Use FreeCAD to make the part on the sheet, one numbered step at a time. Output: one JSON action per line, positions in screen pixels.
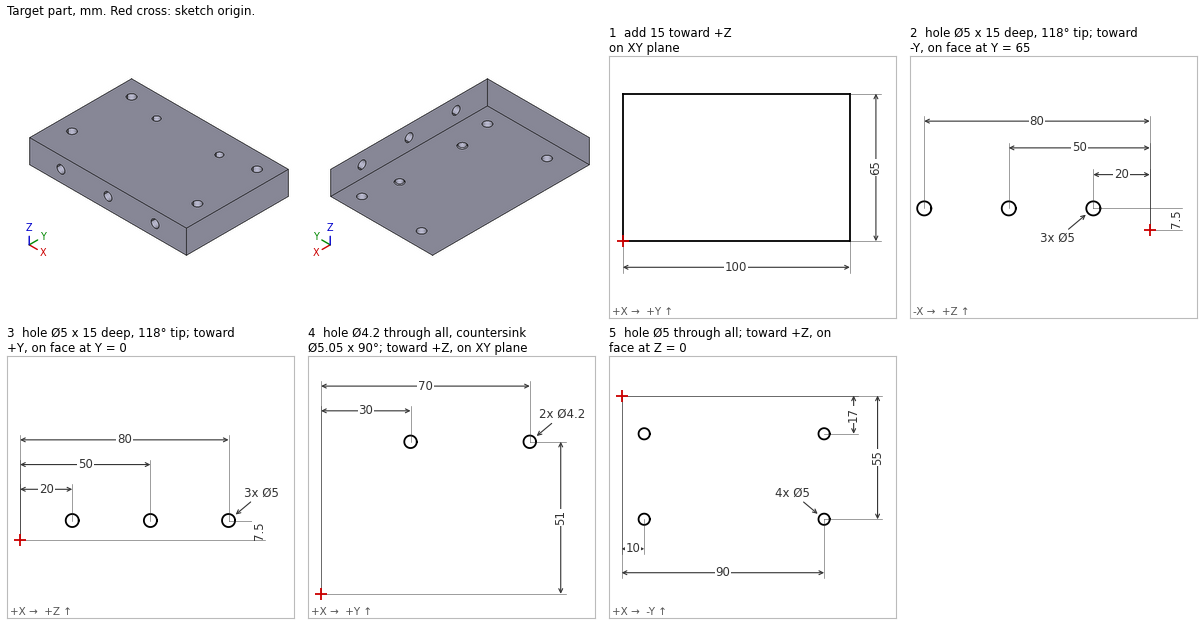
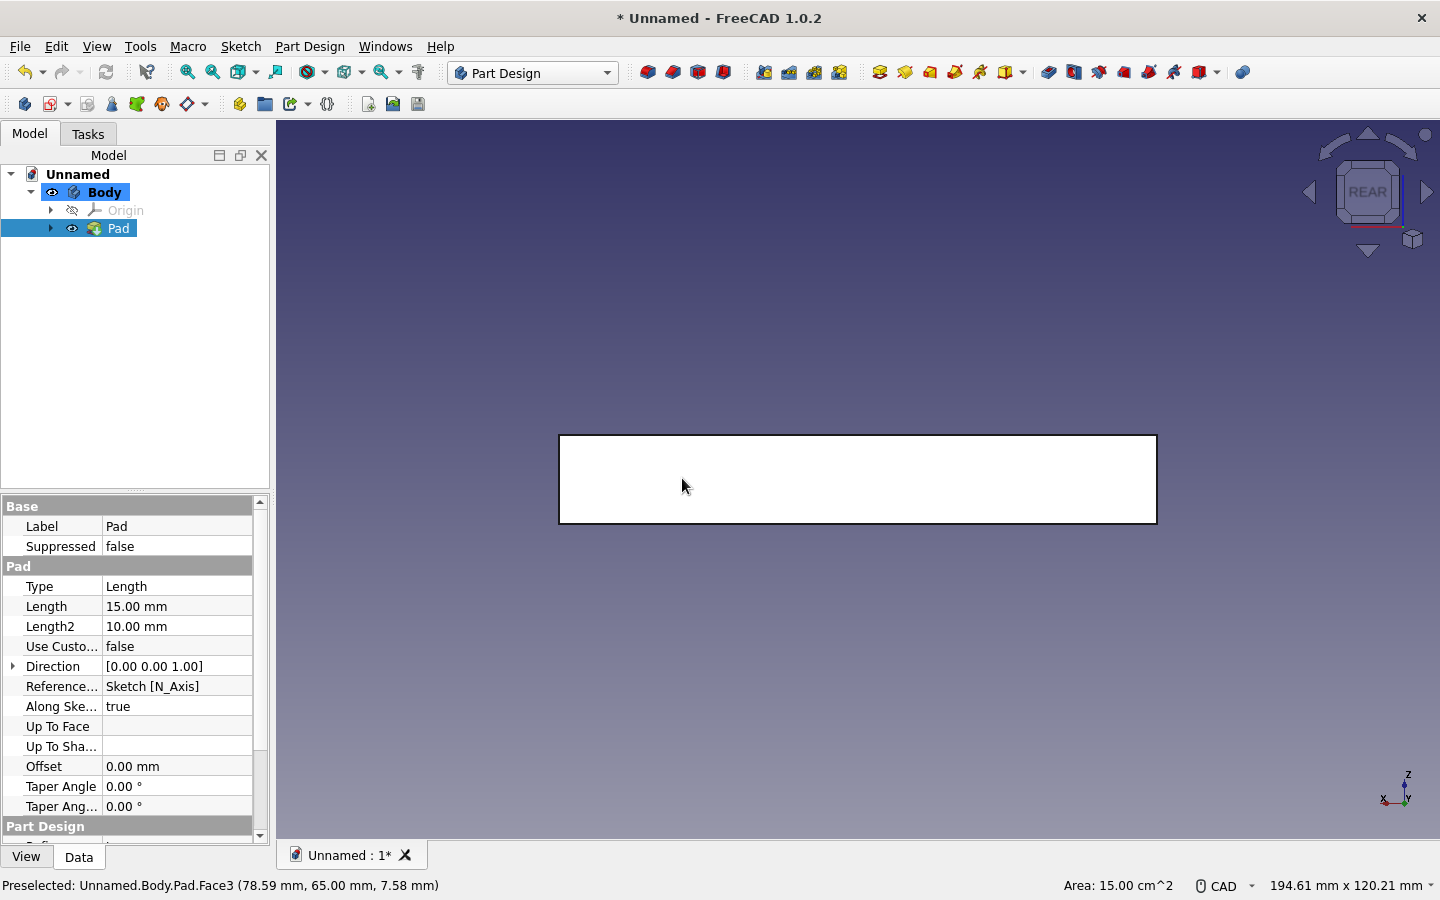
{"action": "left_click", "coordinate": [50, 104]}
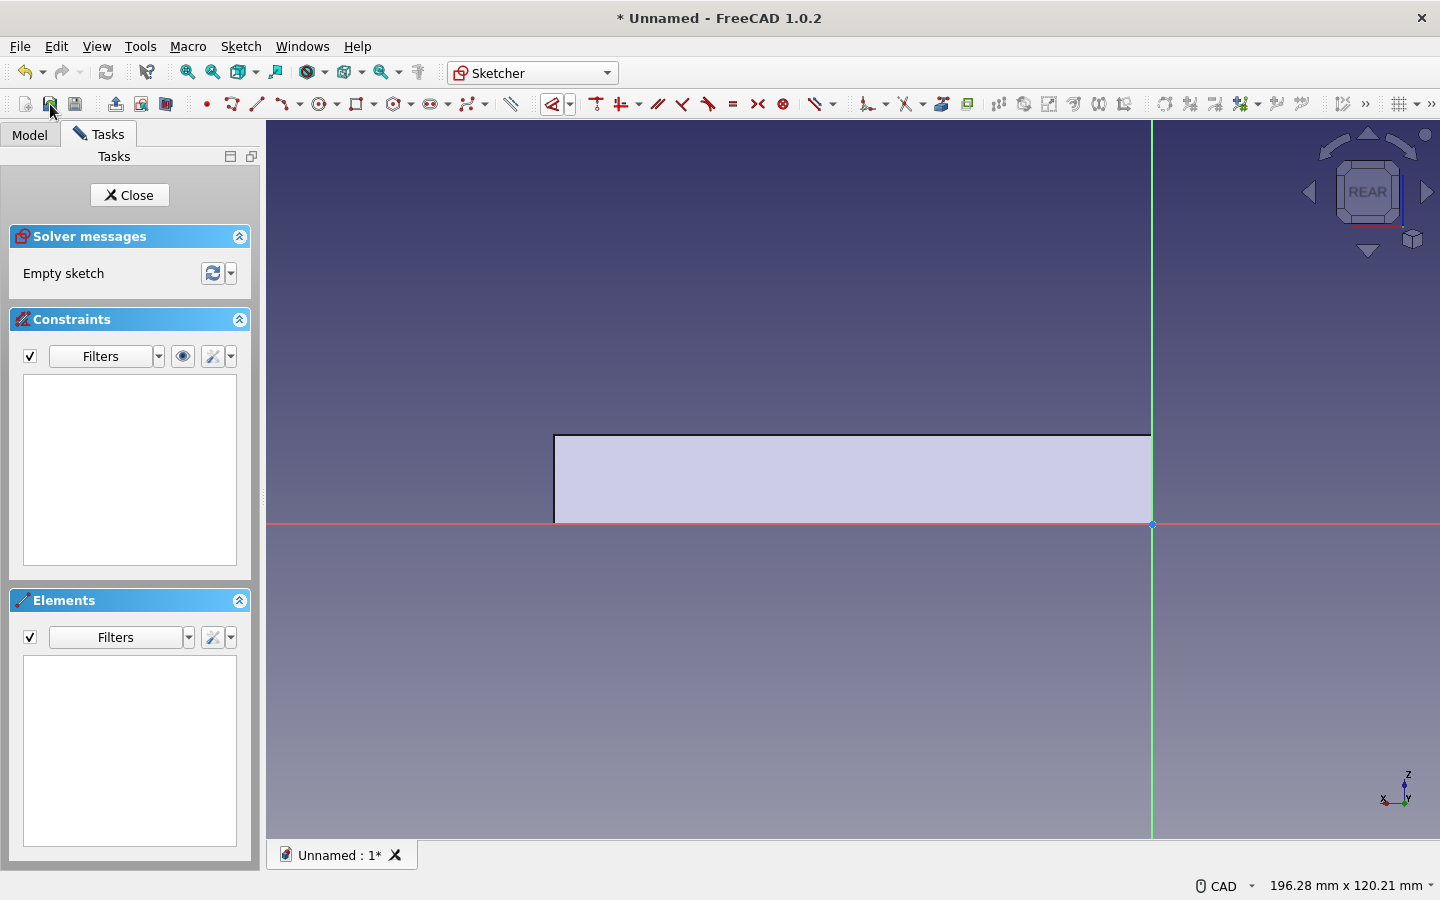
{"action": "scroll", "coordinate": [1151, 525], "scroll_direction": "up", "scroll_amount": 2}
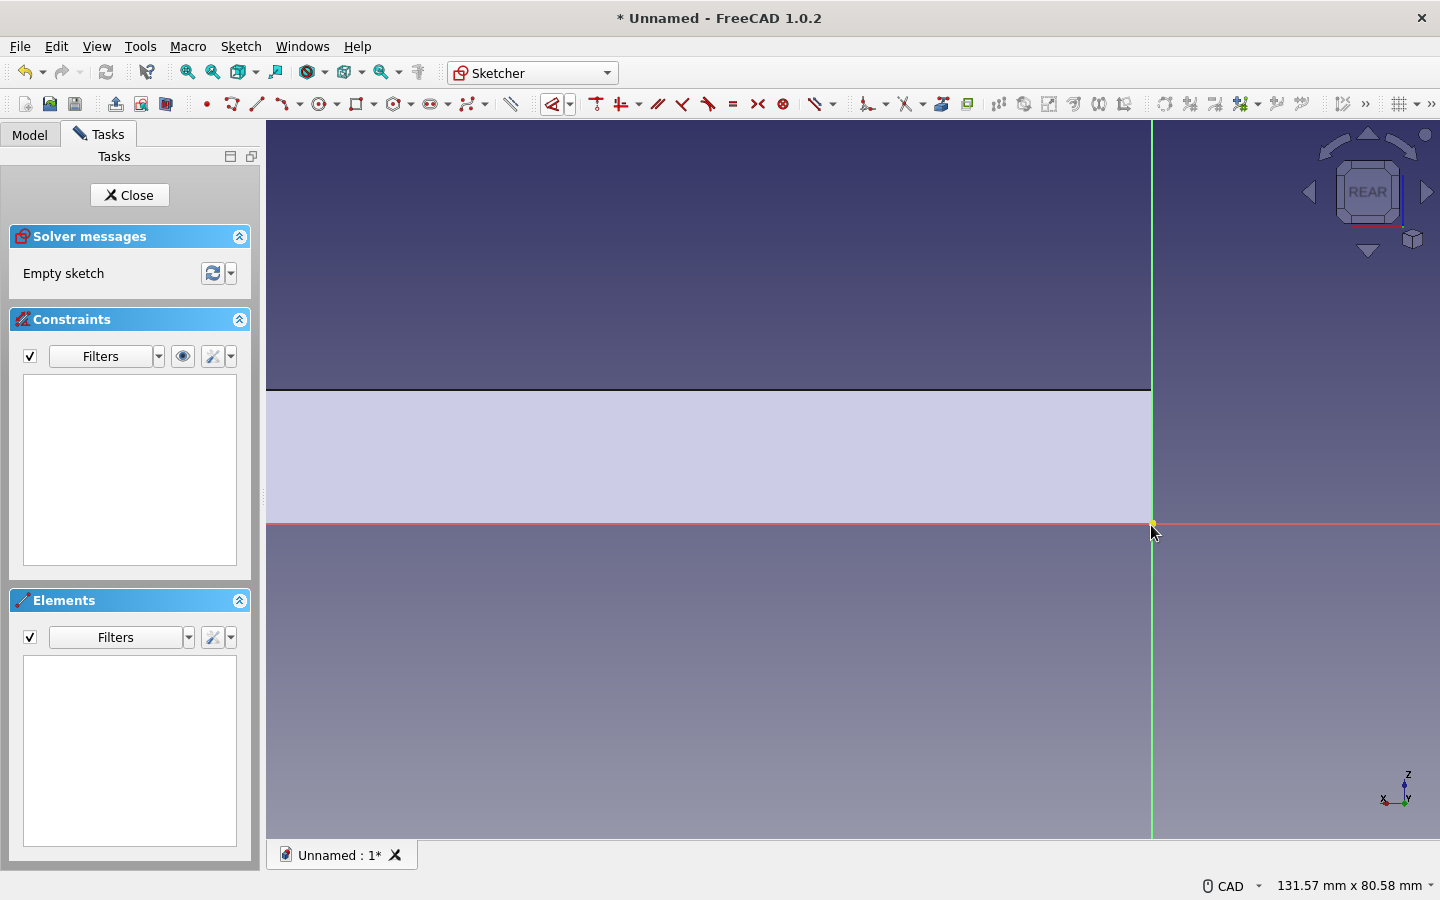
{"action": "left_click", "coordinate": [318, 104]}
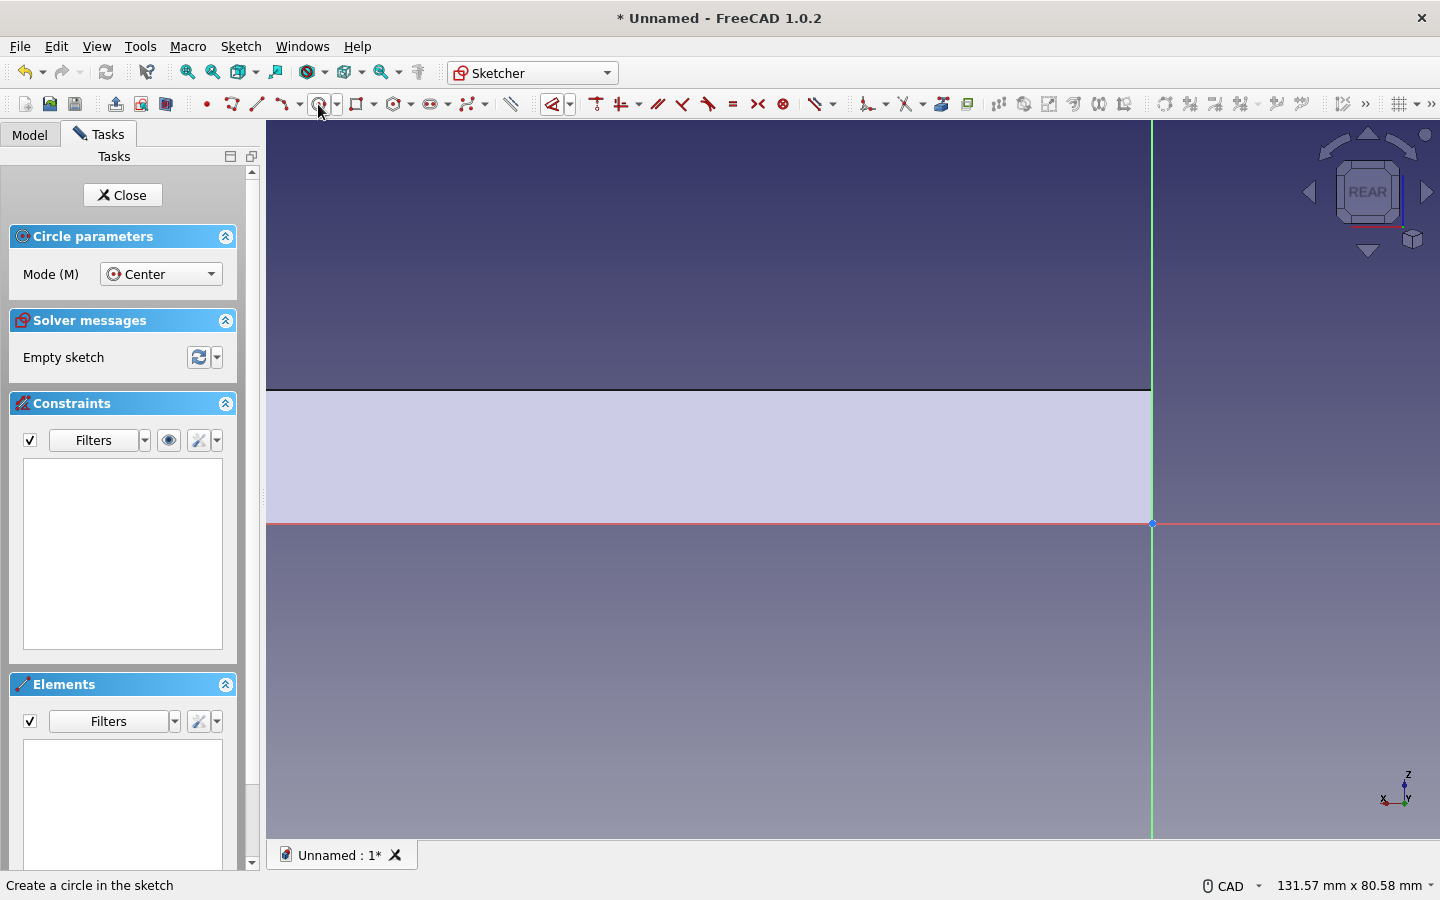
{"action": "left_click", "coordinate": [974, 457]}
{"action": "mouse_move", "coordinate": [990, 441]}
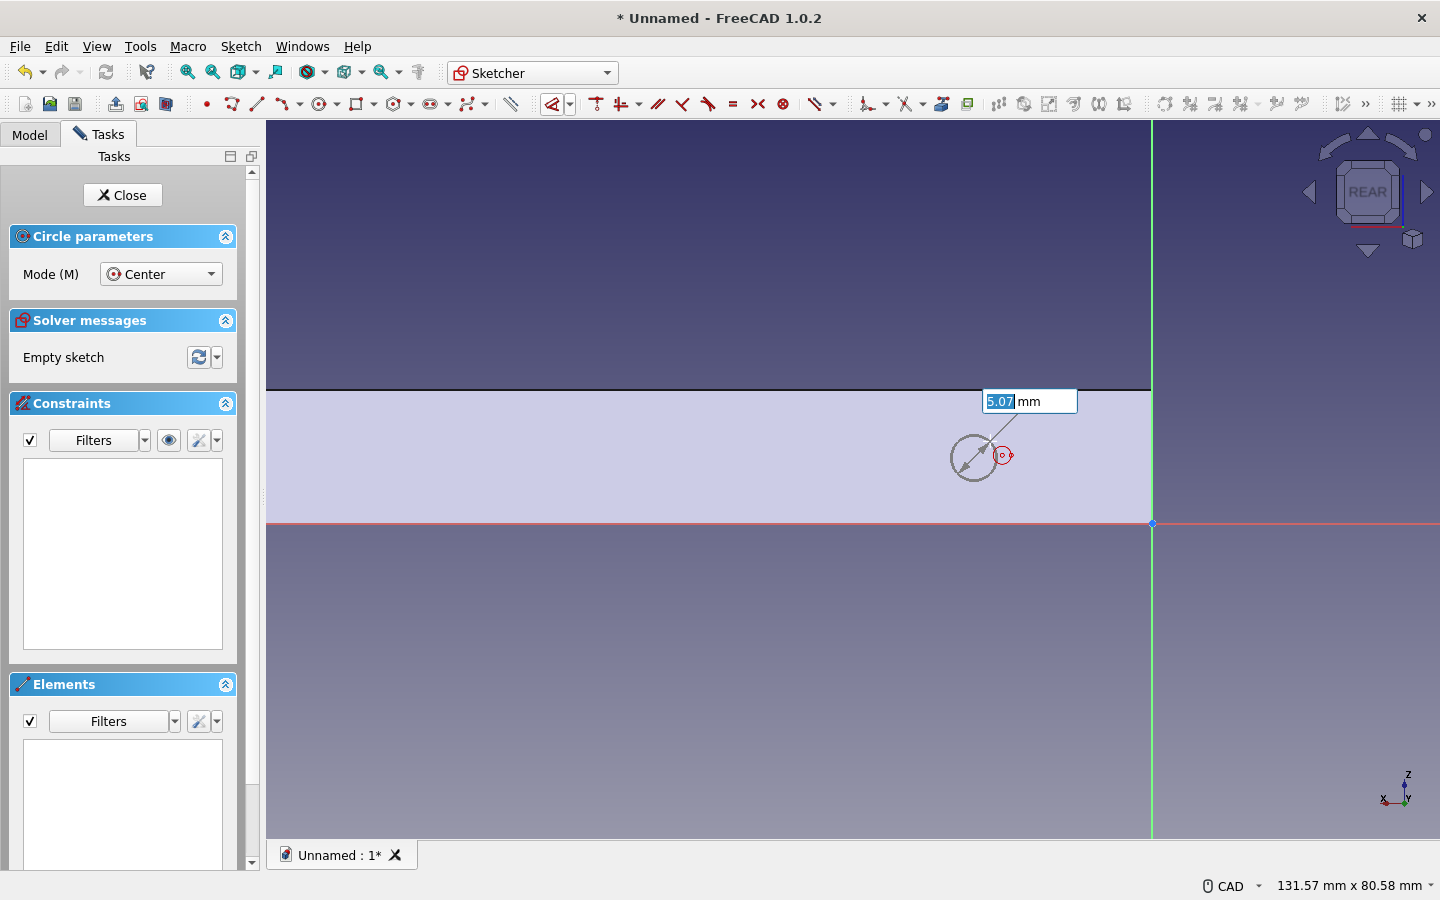
{"action": "type", "text": "5"}
{"action": "key", "text": "Return"}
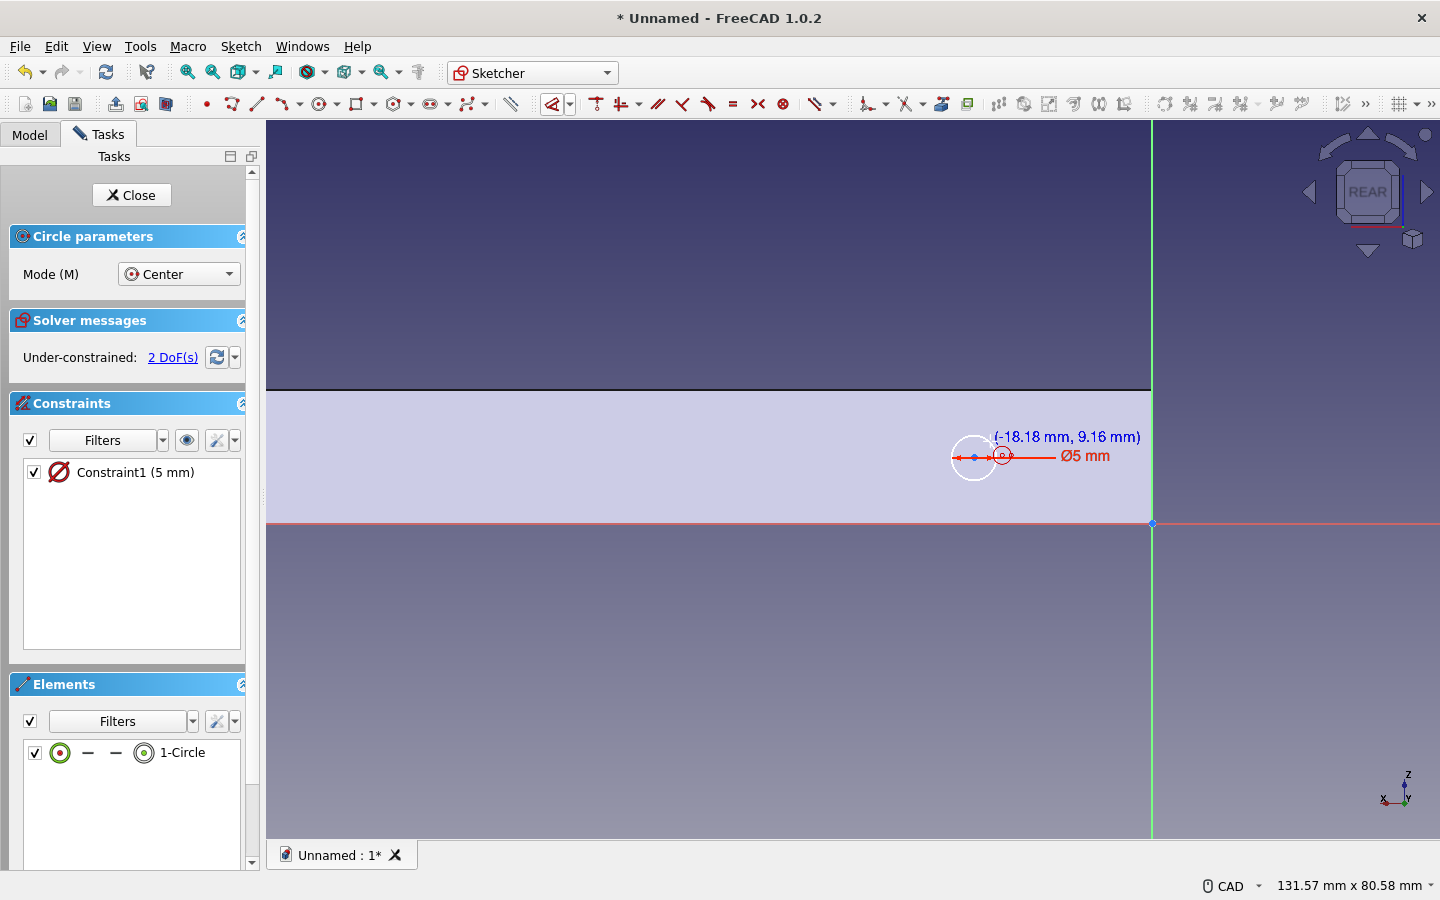
{"action": "left_click", "coordinate": [438, 457]}
{"action": "mouse_move", "coordinate": [454, 441]}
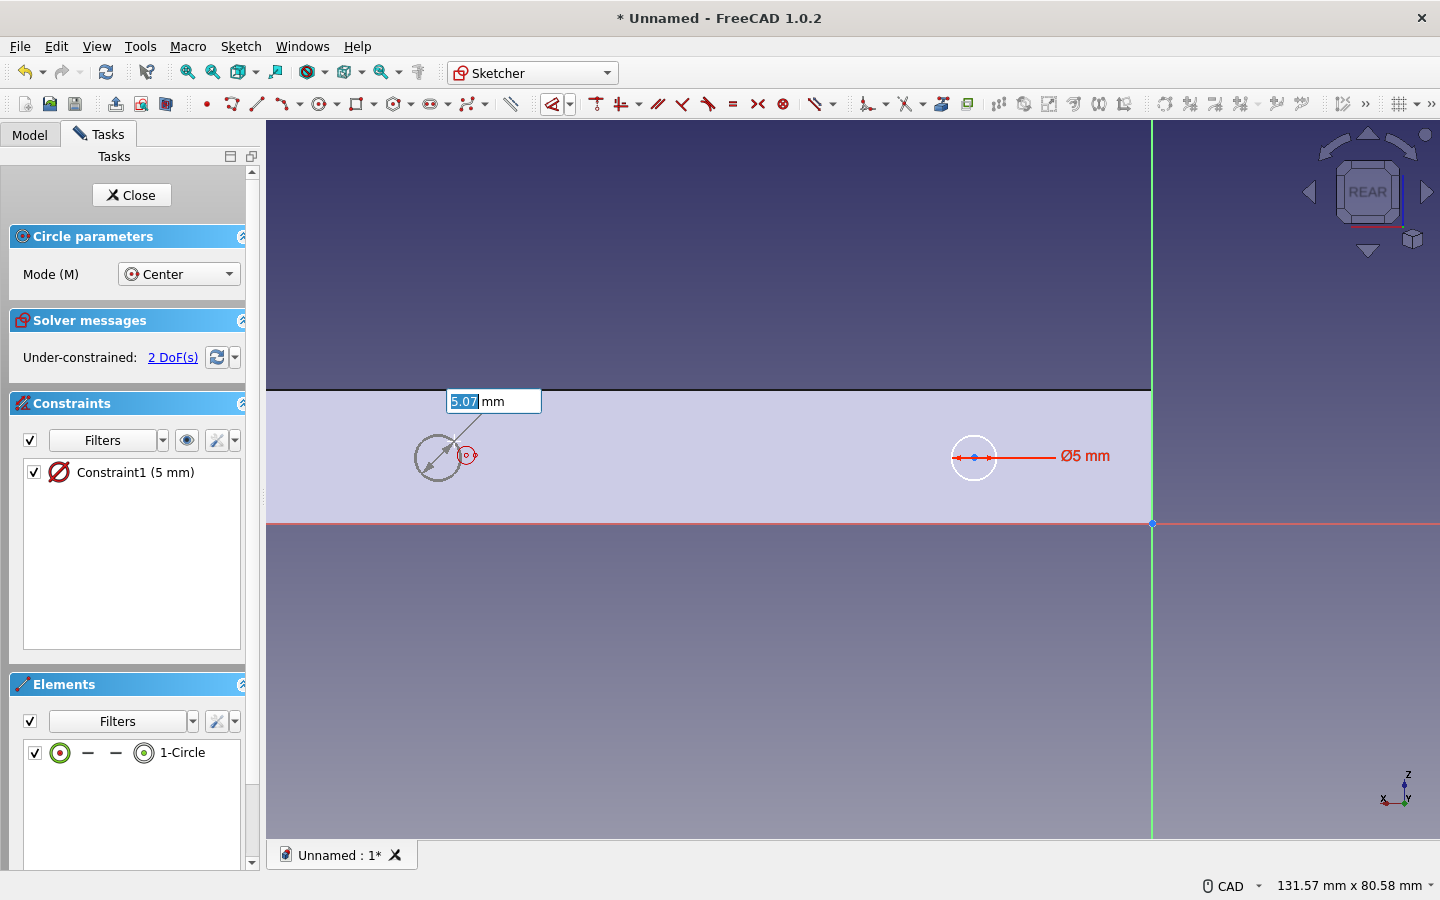
{"action": "type", "text": "5"}
{"action": "key", "text": "Return"}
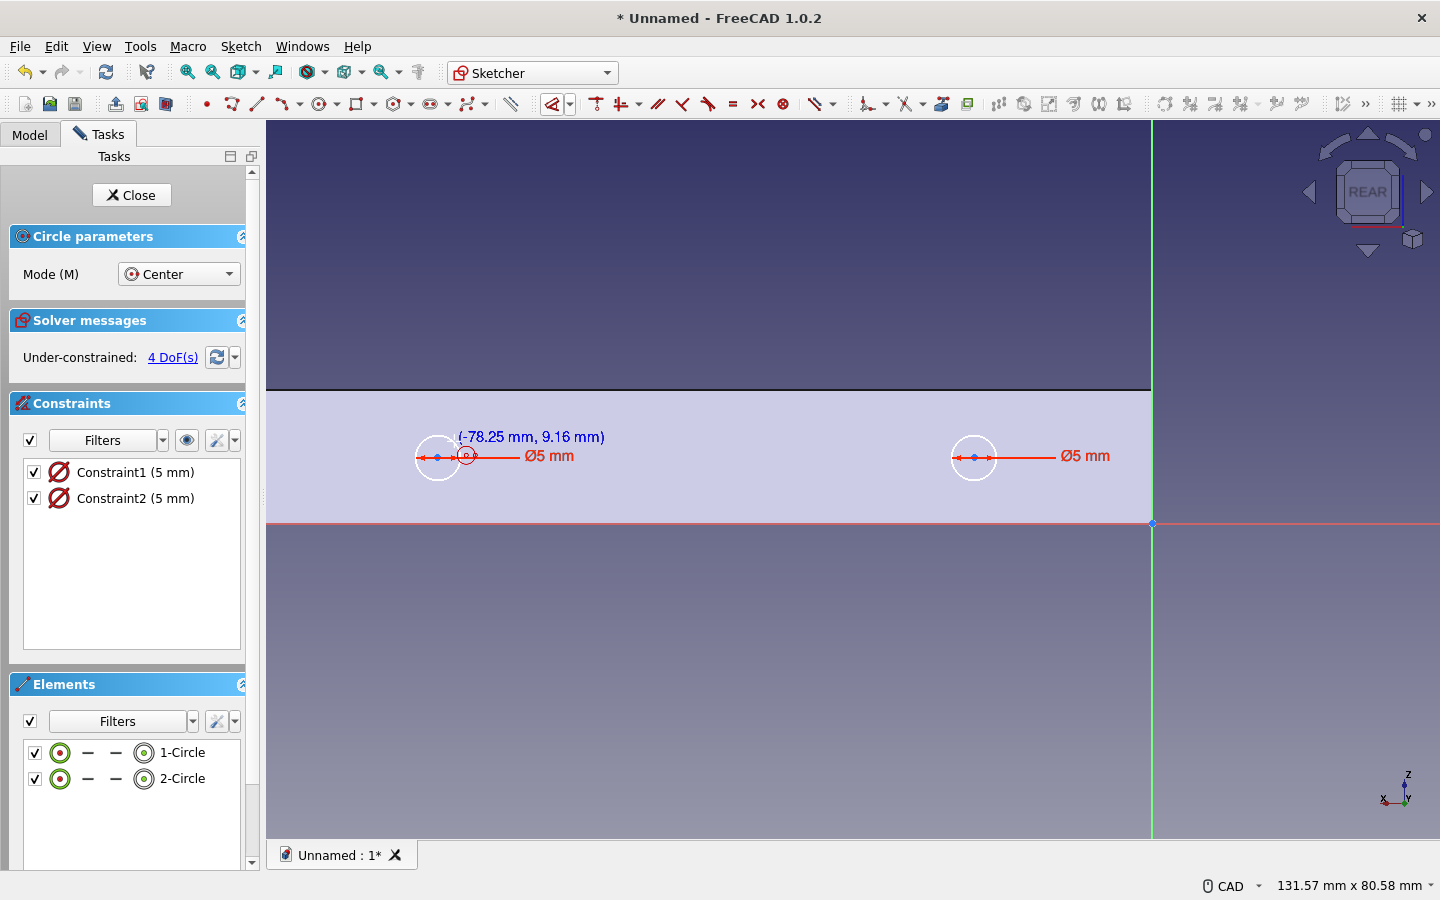
{"action": "left_click", "coordinate": [706, 457]}
{"action": "mouse_move", "coordinate": [722, 441]}